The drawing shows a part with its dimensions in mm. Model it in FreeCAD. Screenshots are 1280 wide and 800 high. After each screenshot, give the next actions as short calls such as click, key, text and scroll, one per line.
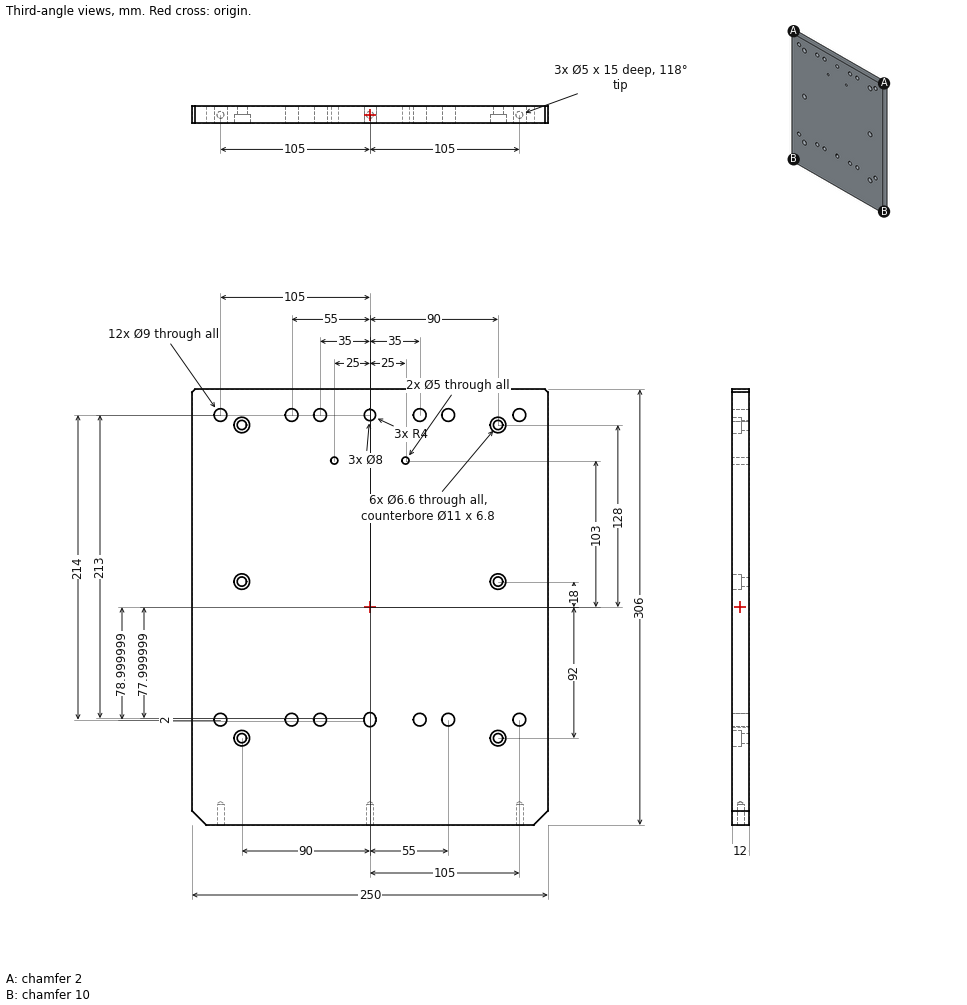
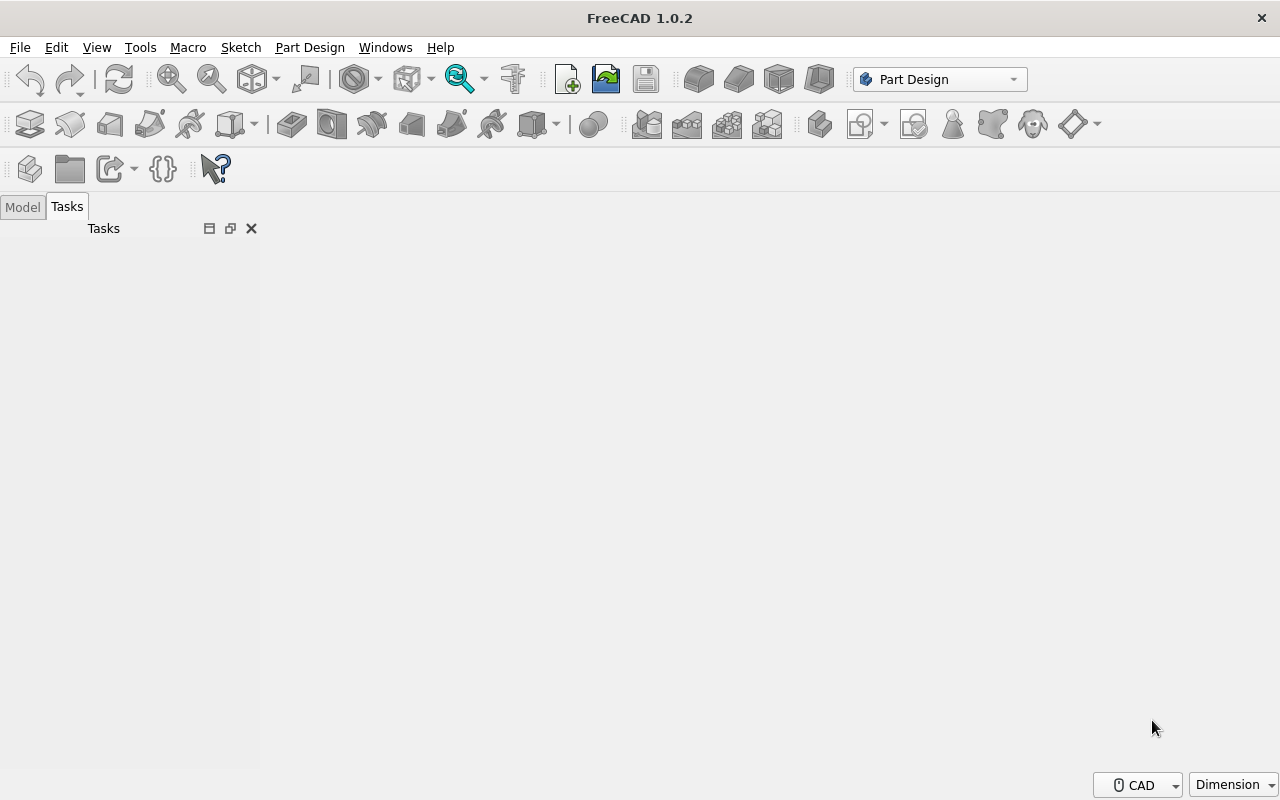
click(566, 80)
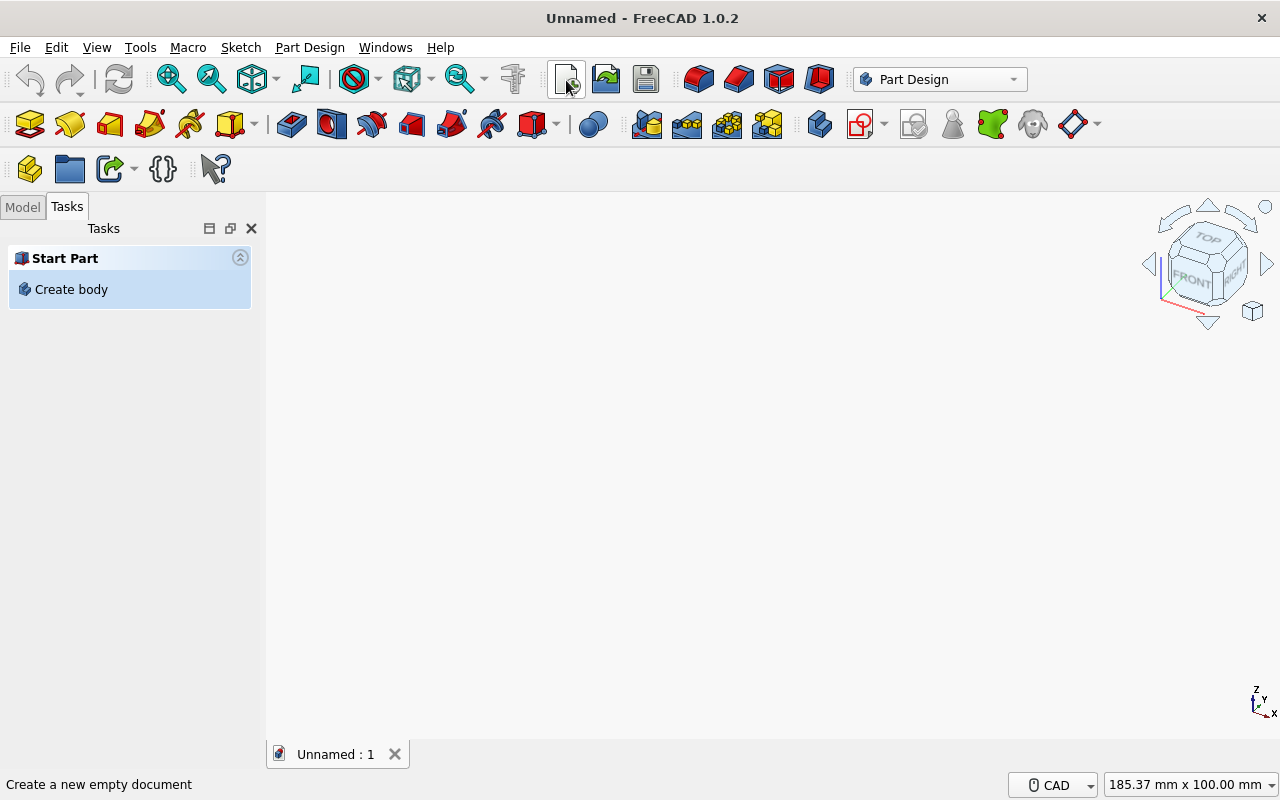
click(860, 124)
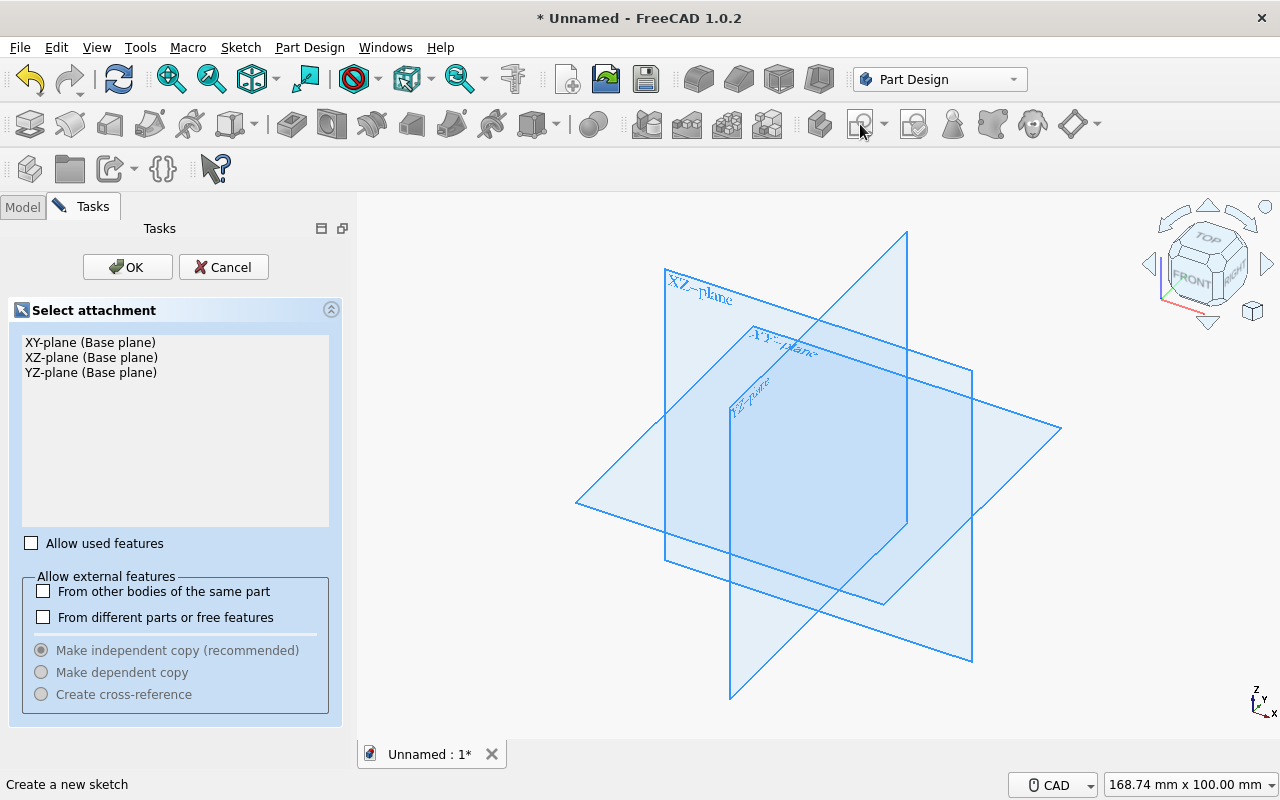
click(82, 358)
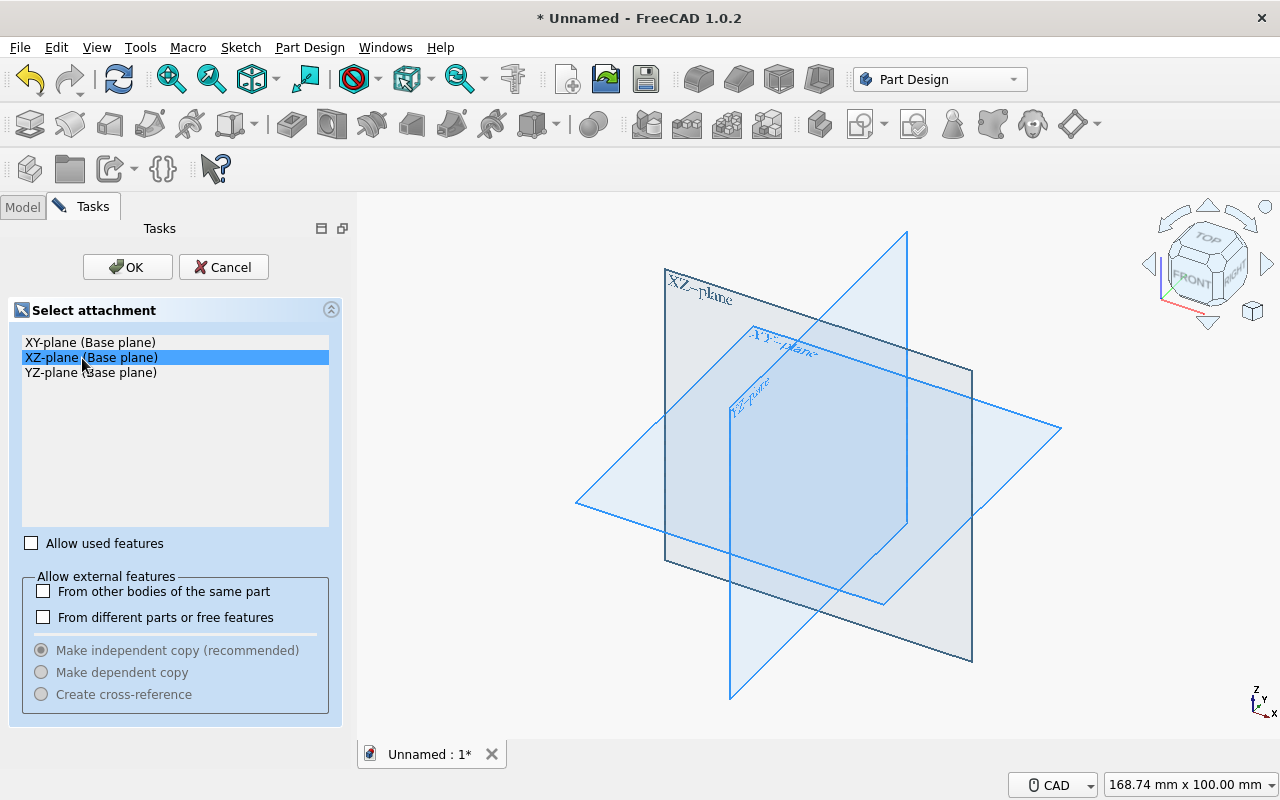
click(128, 267)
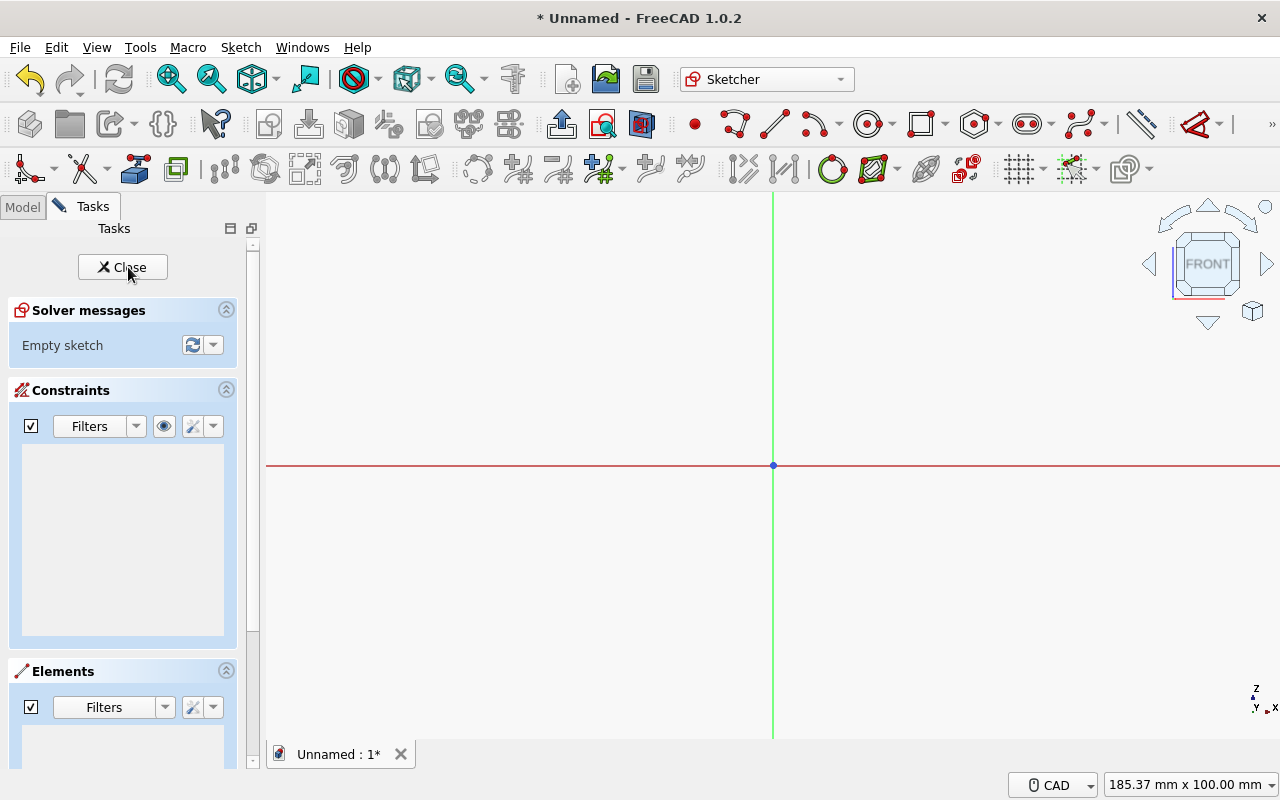
scroll(687, 465, down, 8)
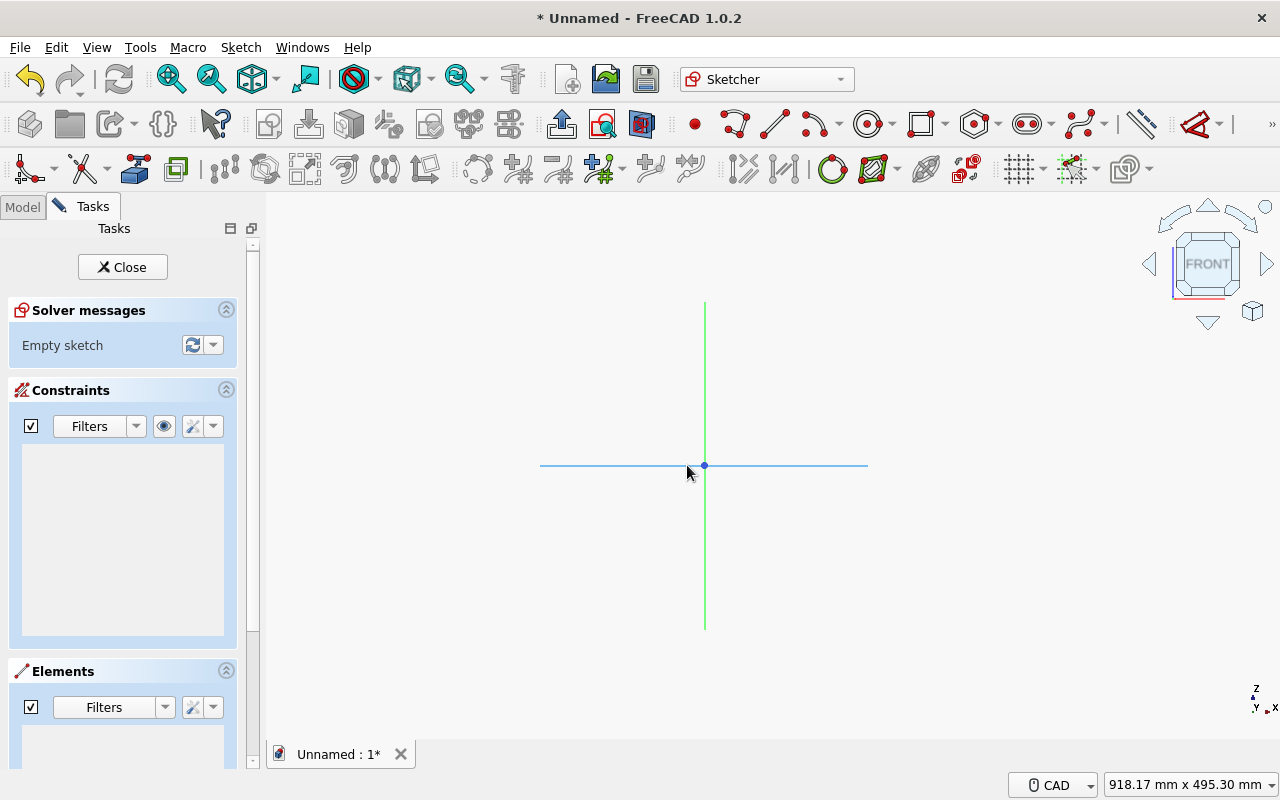
click(948, 124)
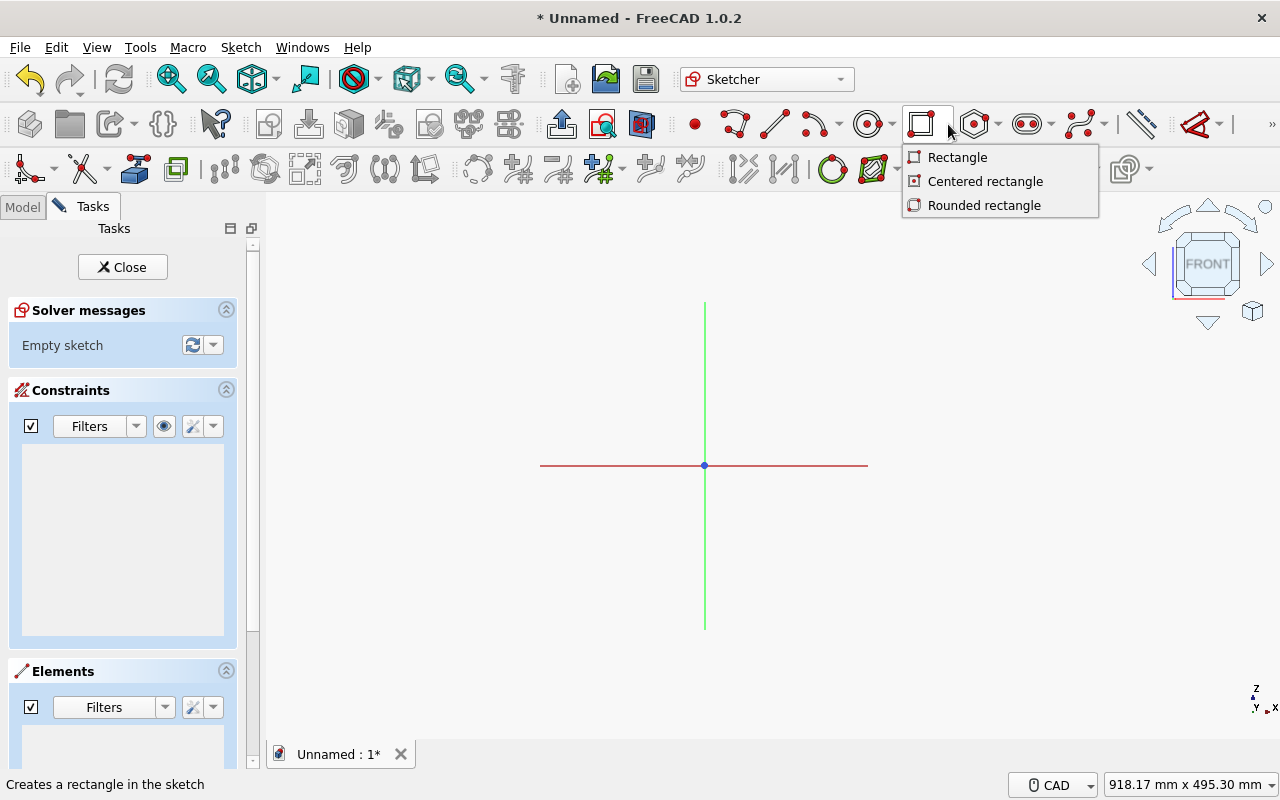
click(1000, 181)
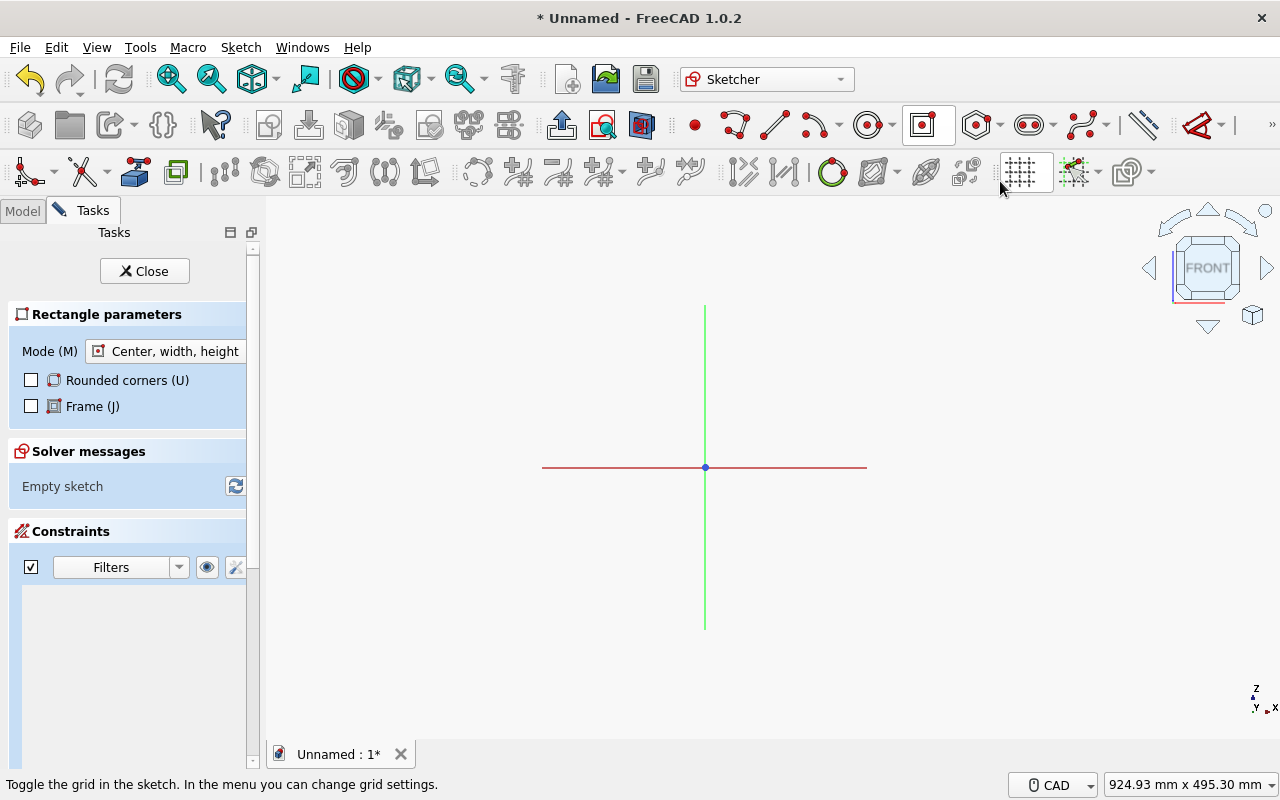
click(705, 468)
move(842, 300)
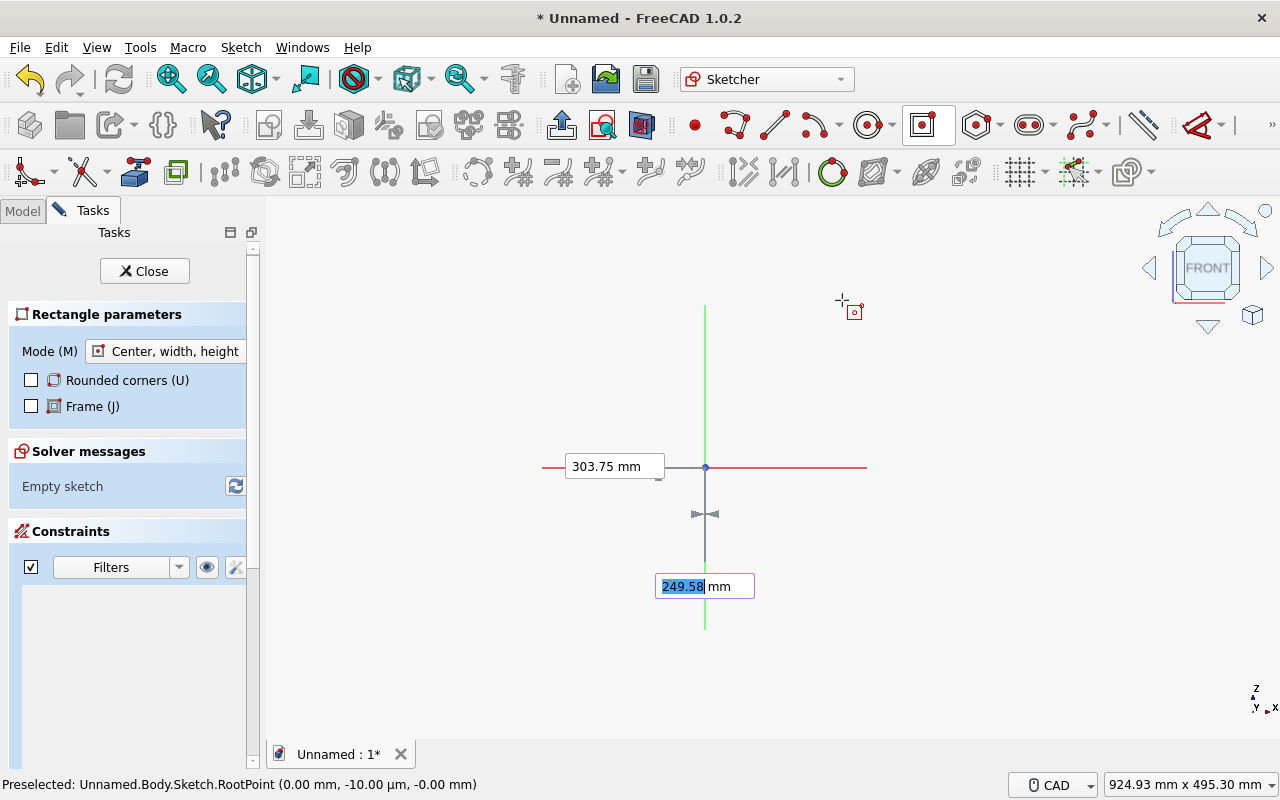
text(250)
key(Tab)
text(306)
key(Return)
key(Escape)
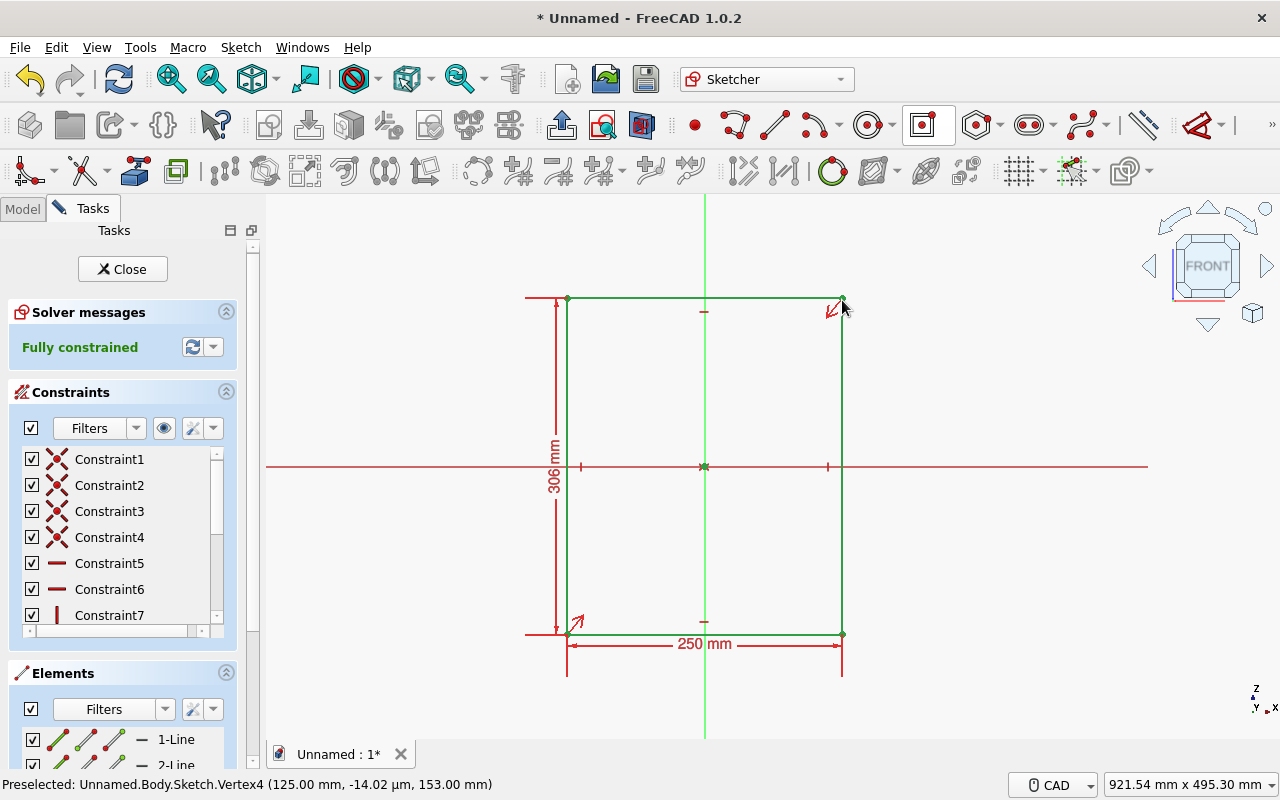
click(123, 269)